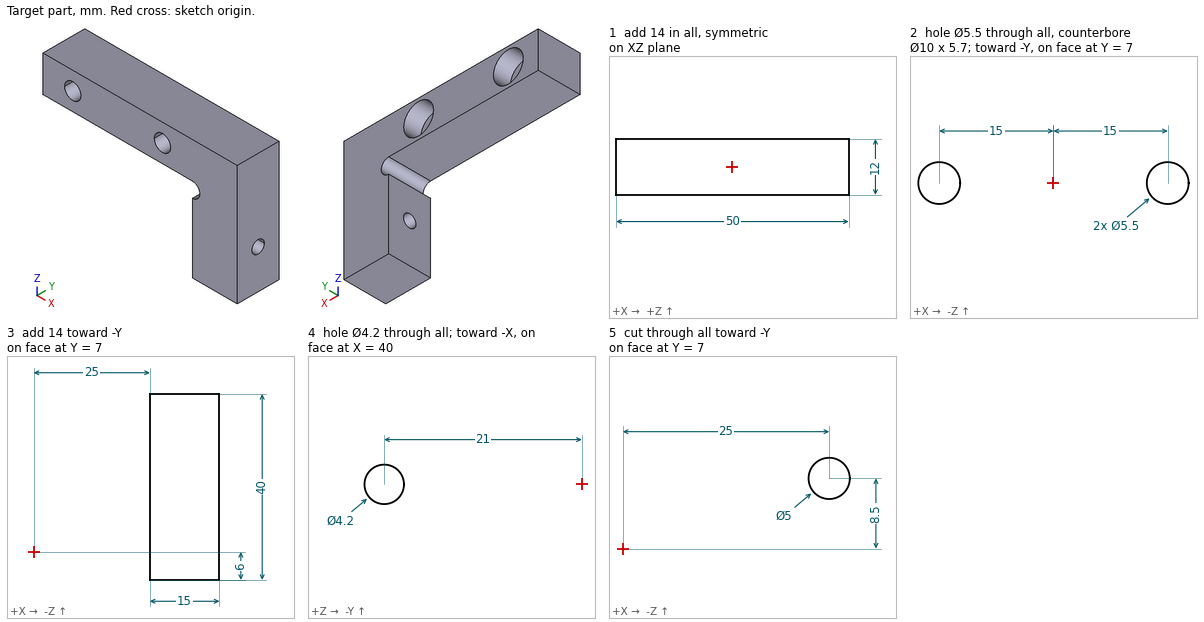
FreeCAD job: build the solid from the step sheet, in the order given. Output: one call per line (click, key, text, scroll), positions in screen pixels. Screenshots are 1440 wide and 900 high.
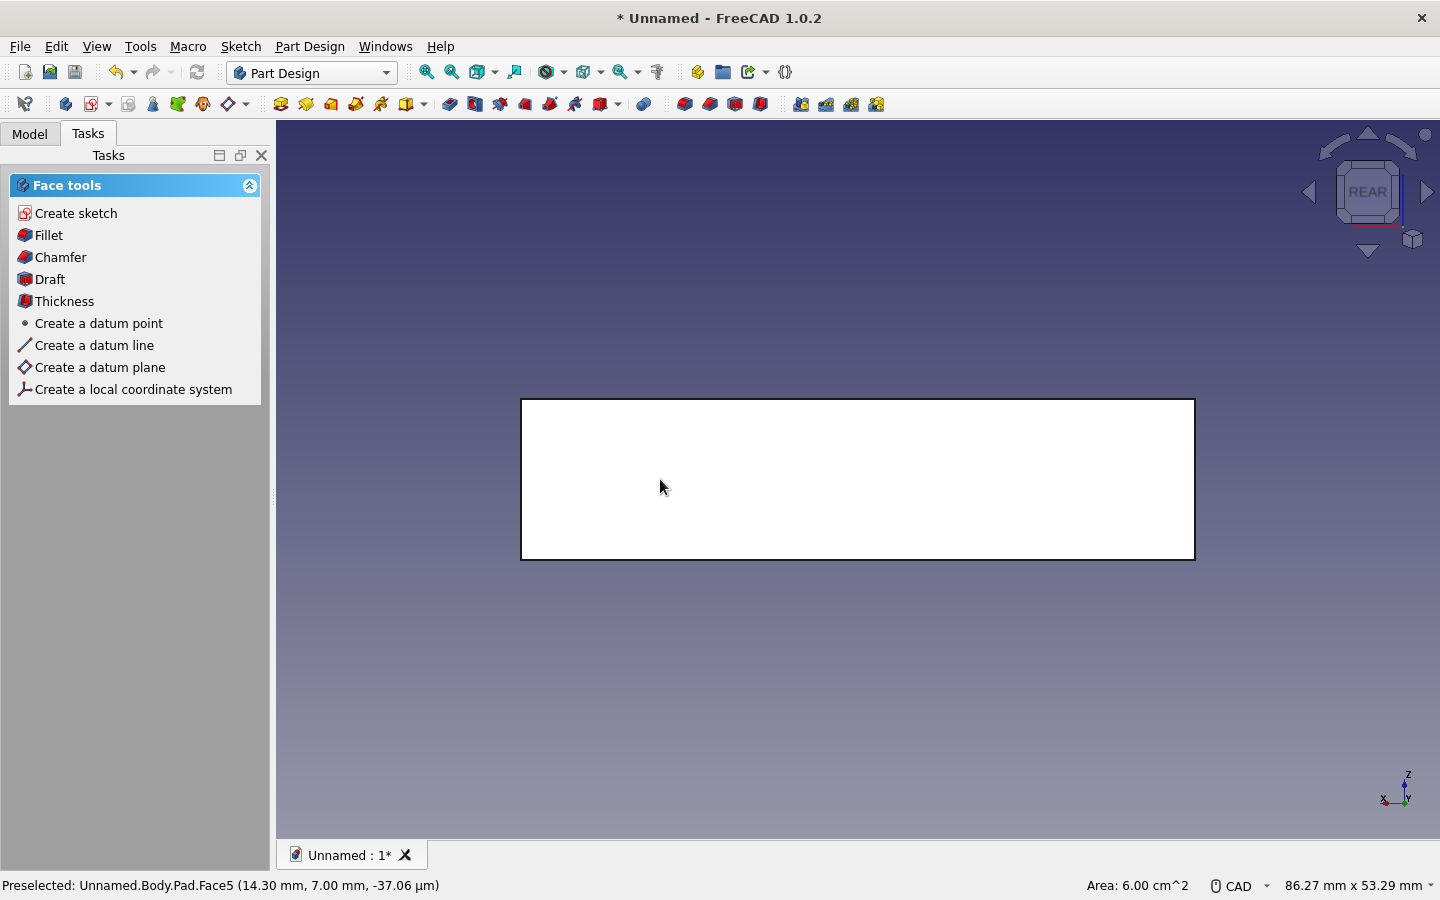
click(90, 104)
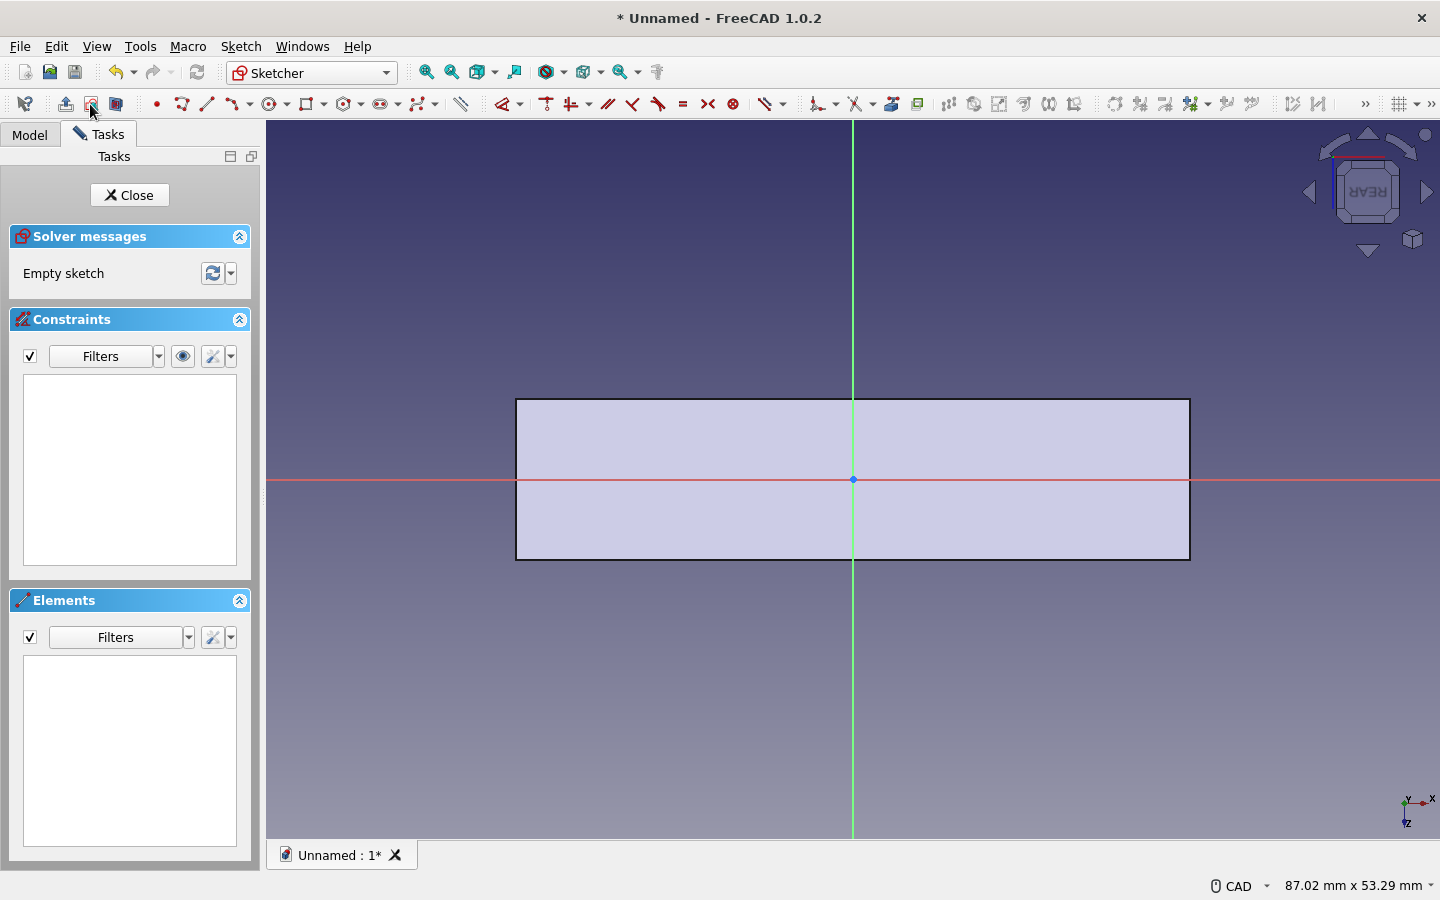
scroll(992, 479, up, 2)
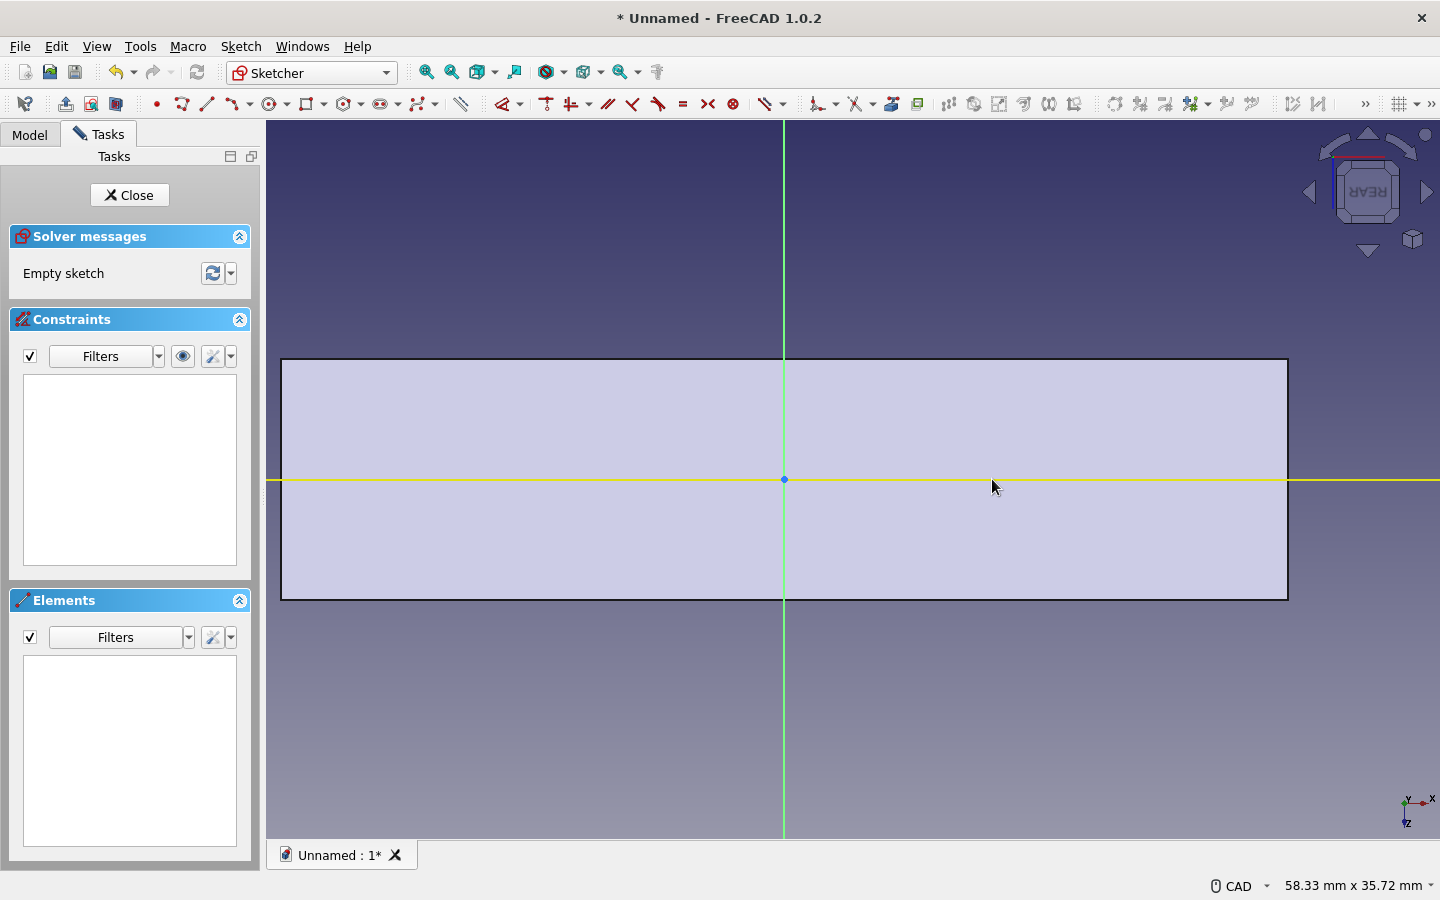
click(268, 104)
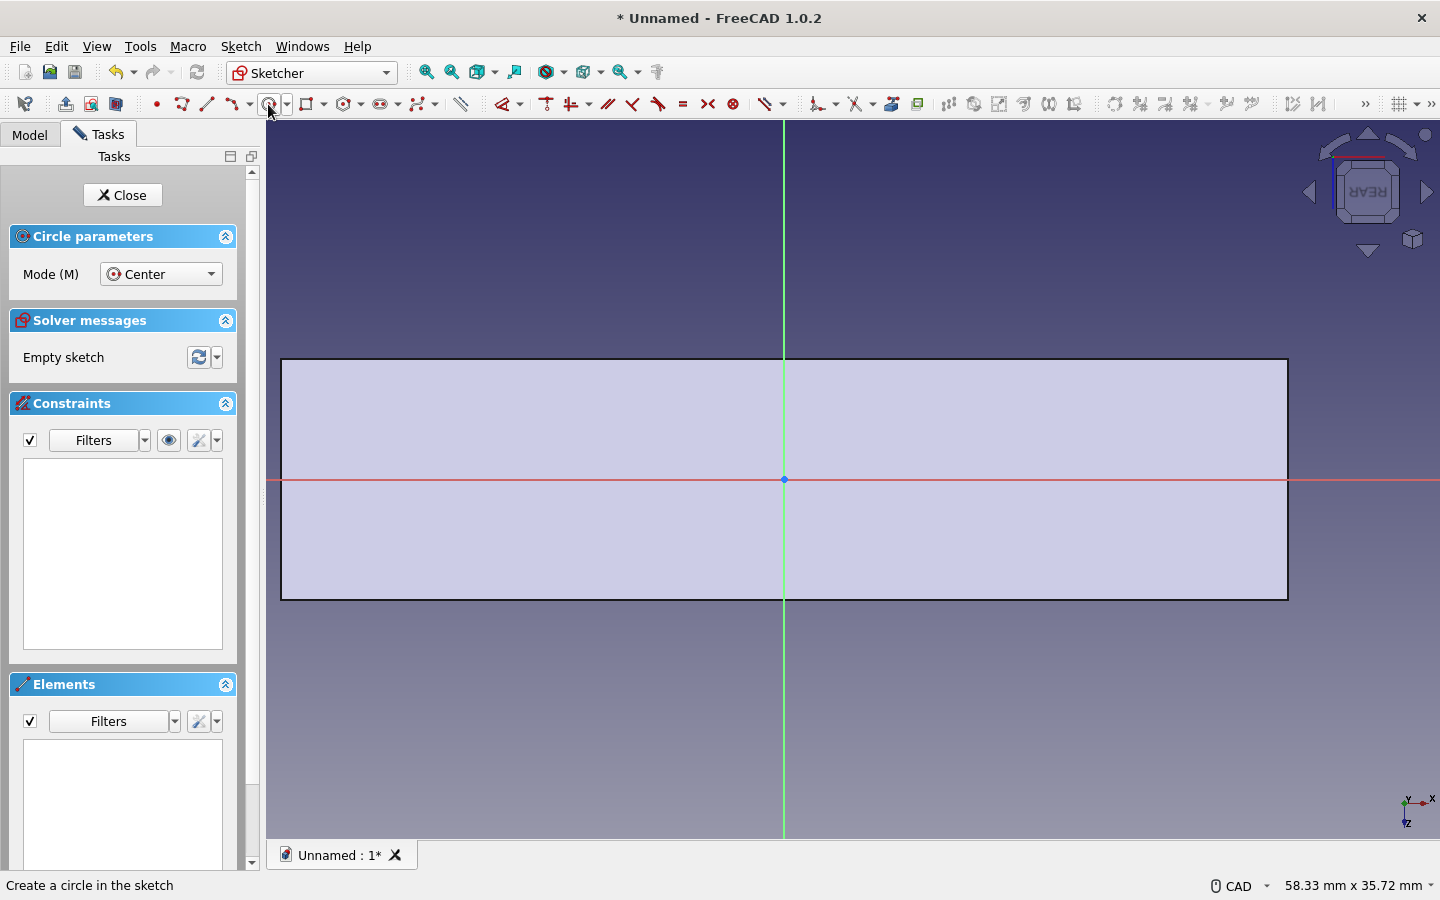
click(1086, 479)
move(1125, 440)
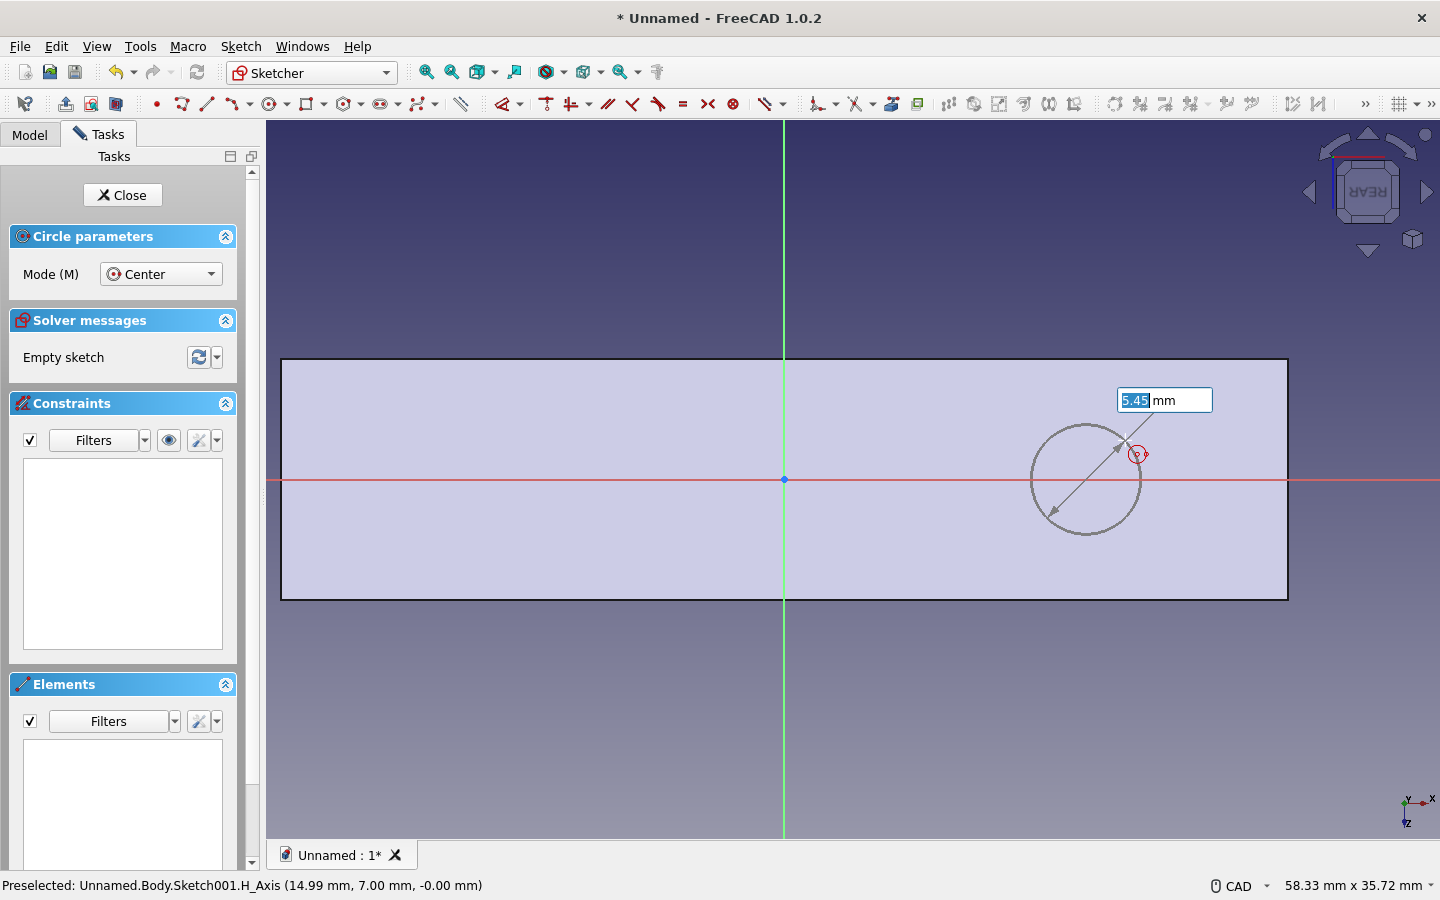
text(5.5)
key(Return)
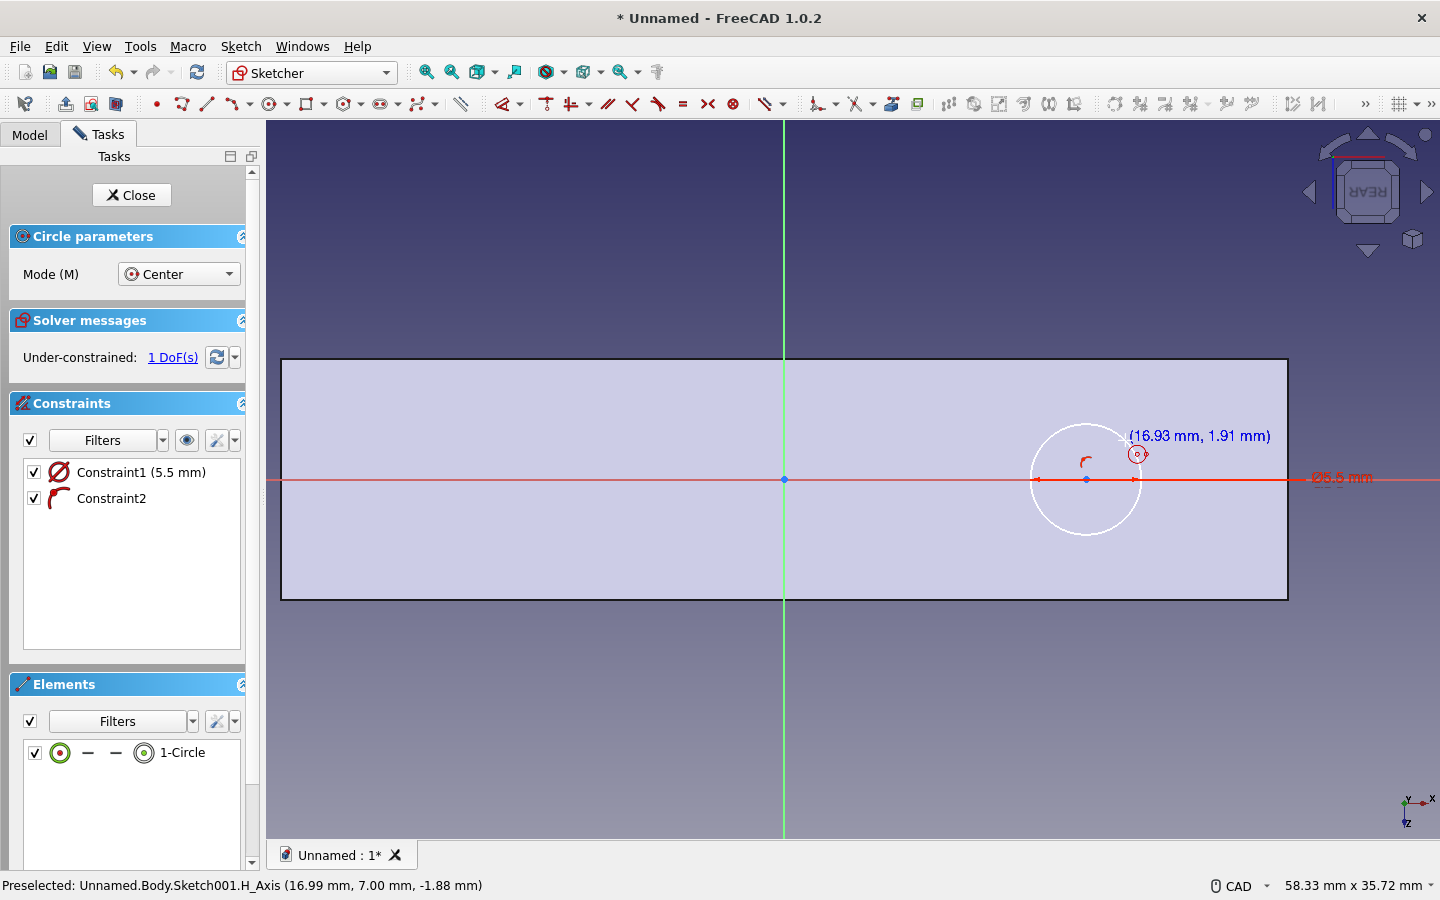
click(482, 479)
move(522, 440)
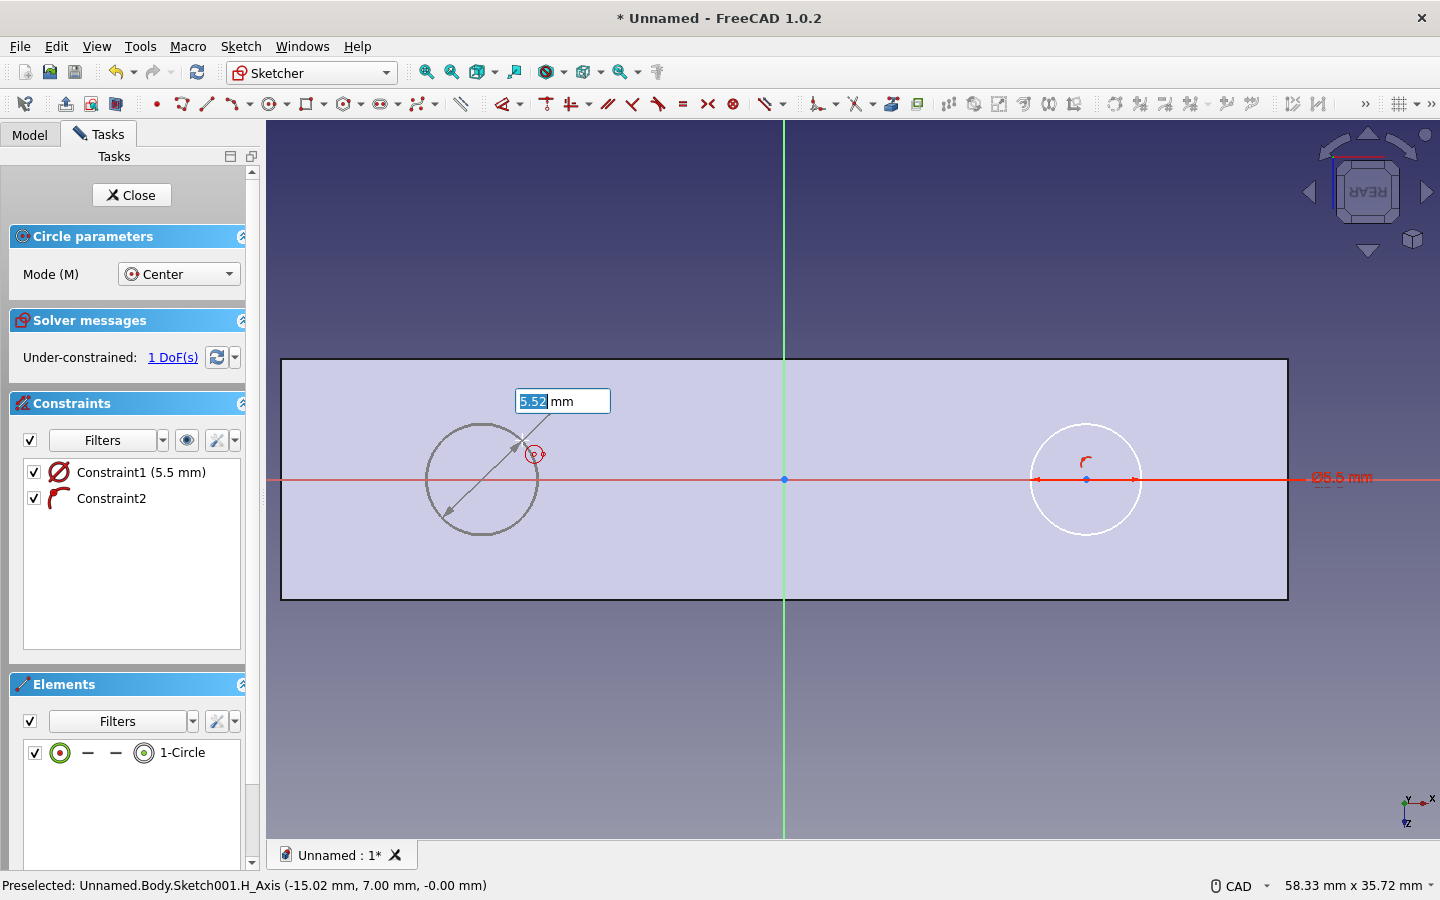
text(5.5)
key(Return)
key(Escape)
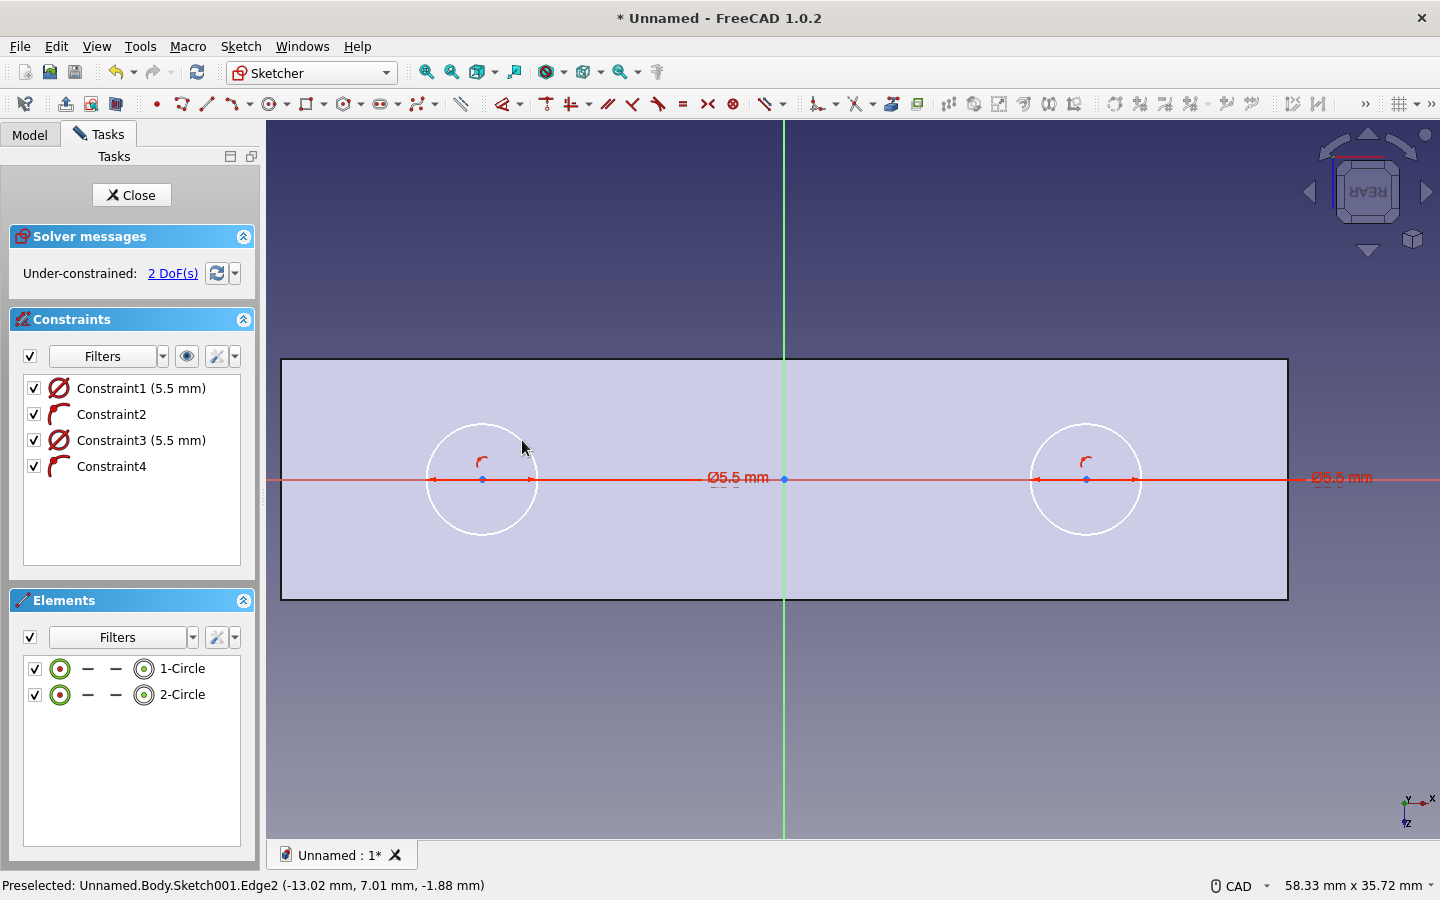
click(502, 104)